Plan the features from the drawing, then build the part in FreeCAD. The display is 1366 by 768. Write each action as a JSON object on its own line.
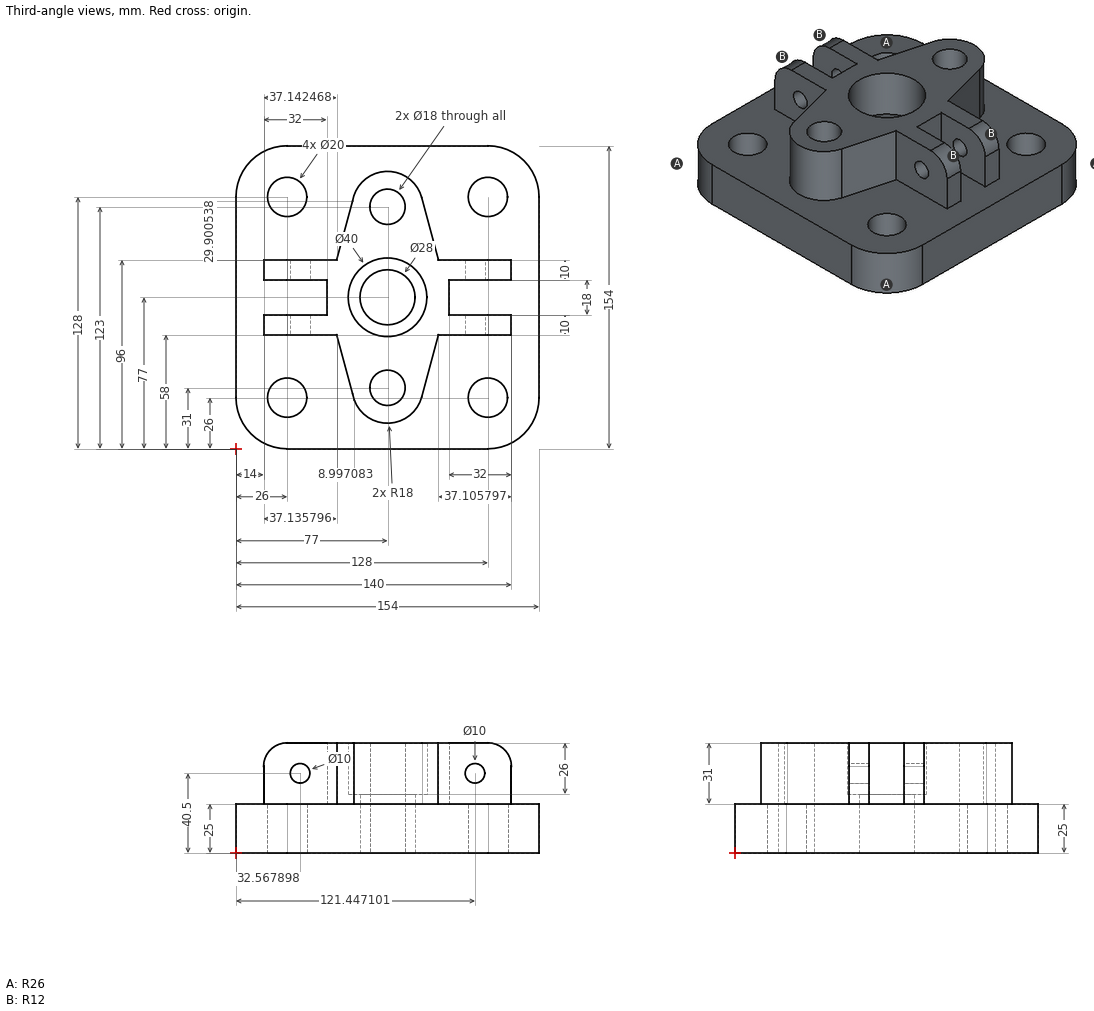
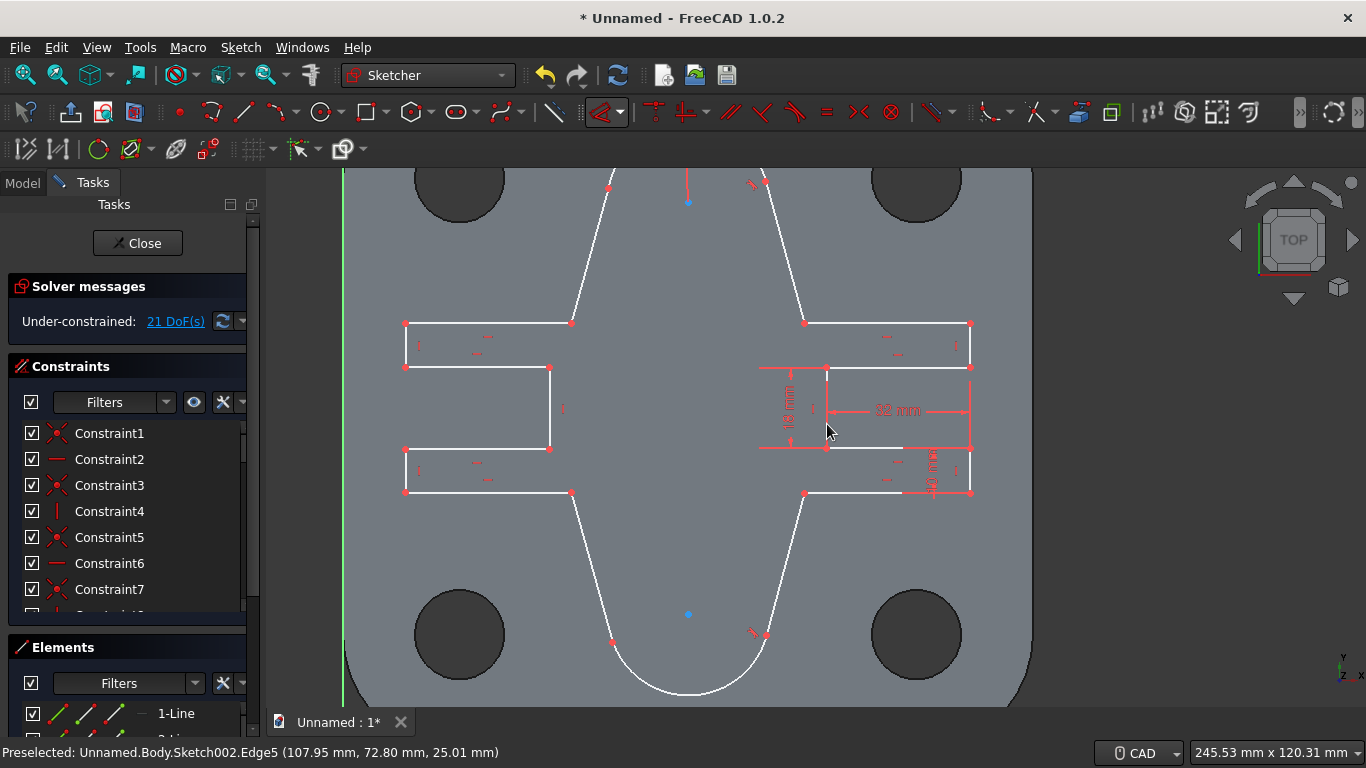
{"action": "left_click", "coordinate": [870, 368]}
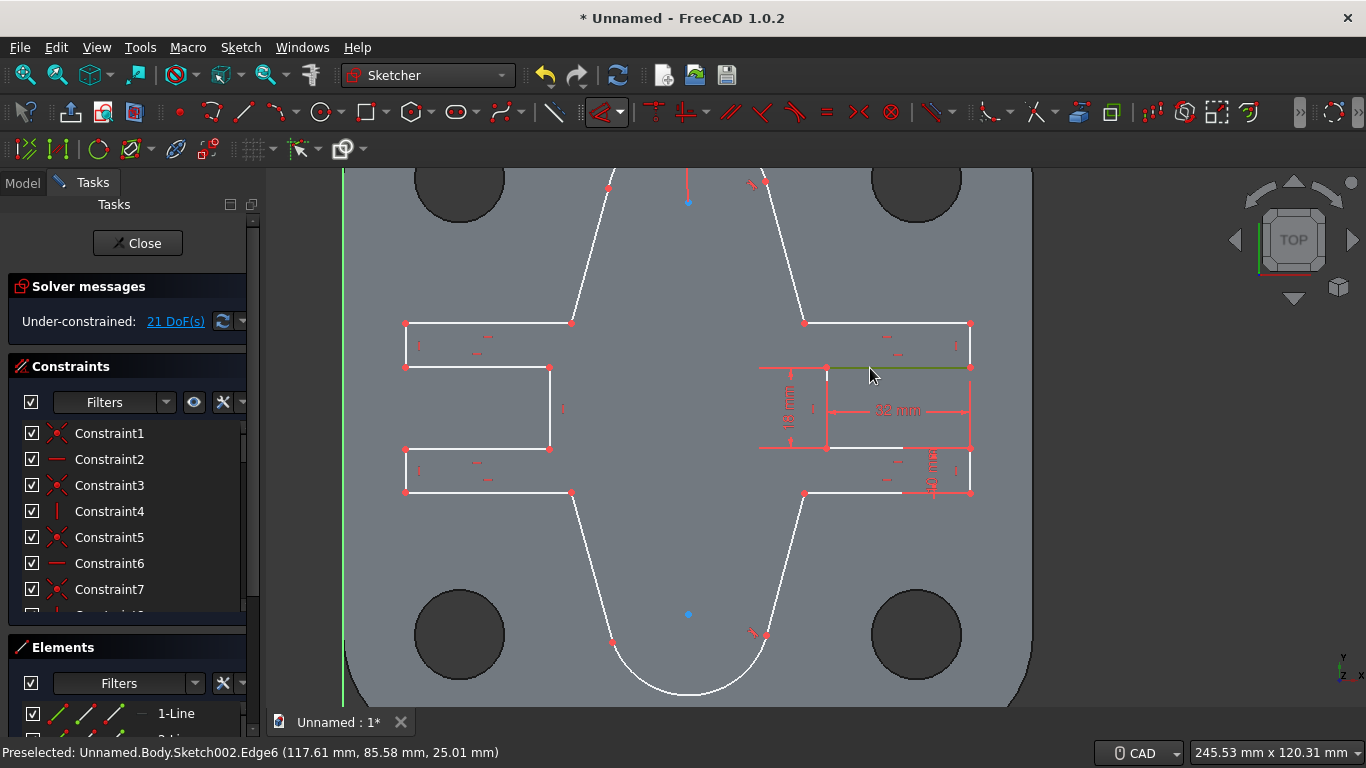
{"action": "key", "text": "l"}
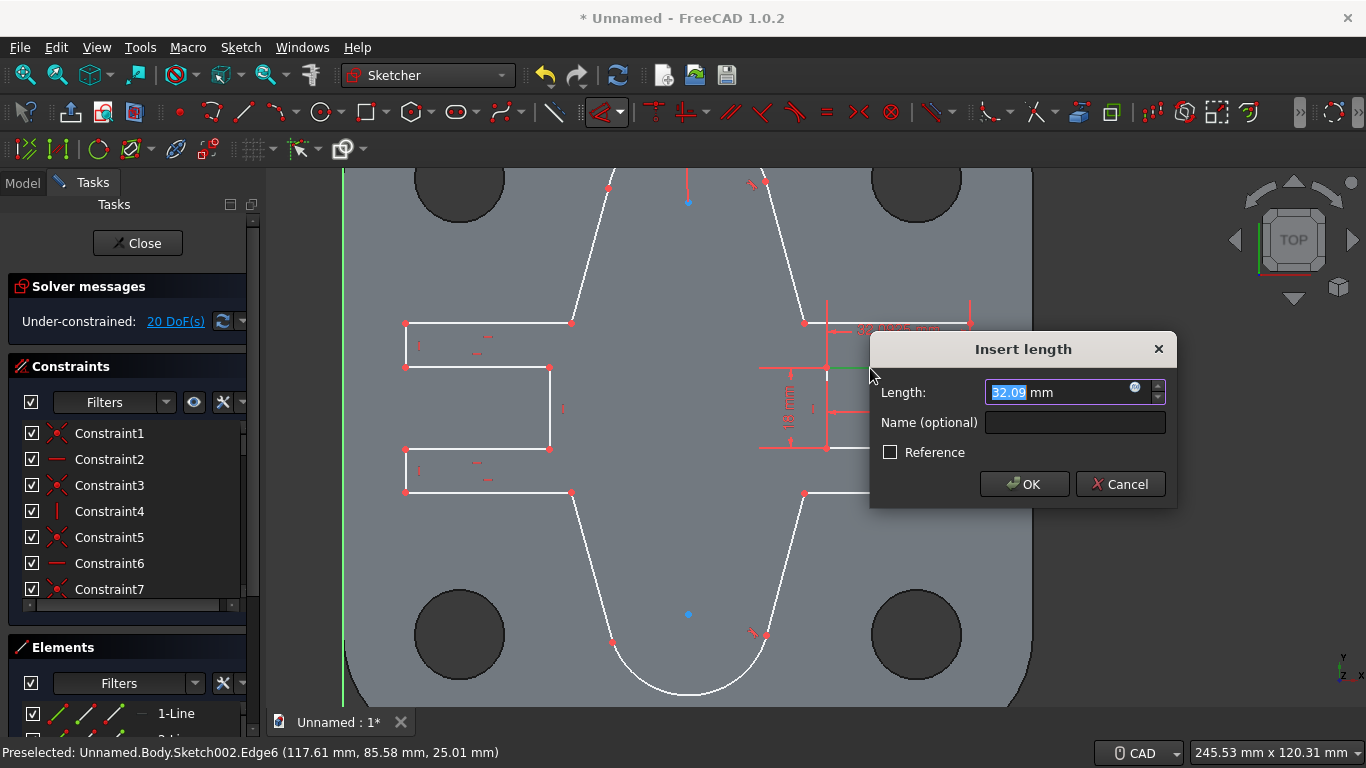
{"action": "type", "text": "32"}
{"action": "key", "text": "Return"}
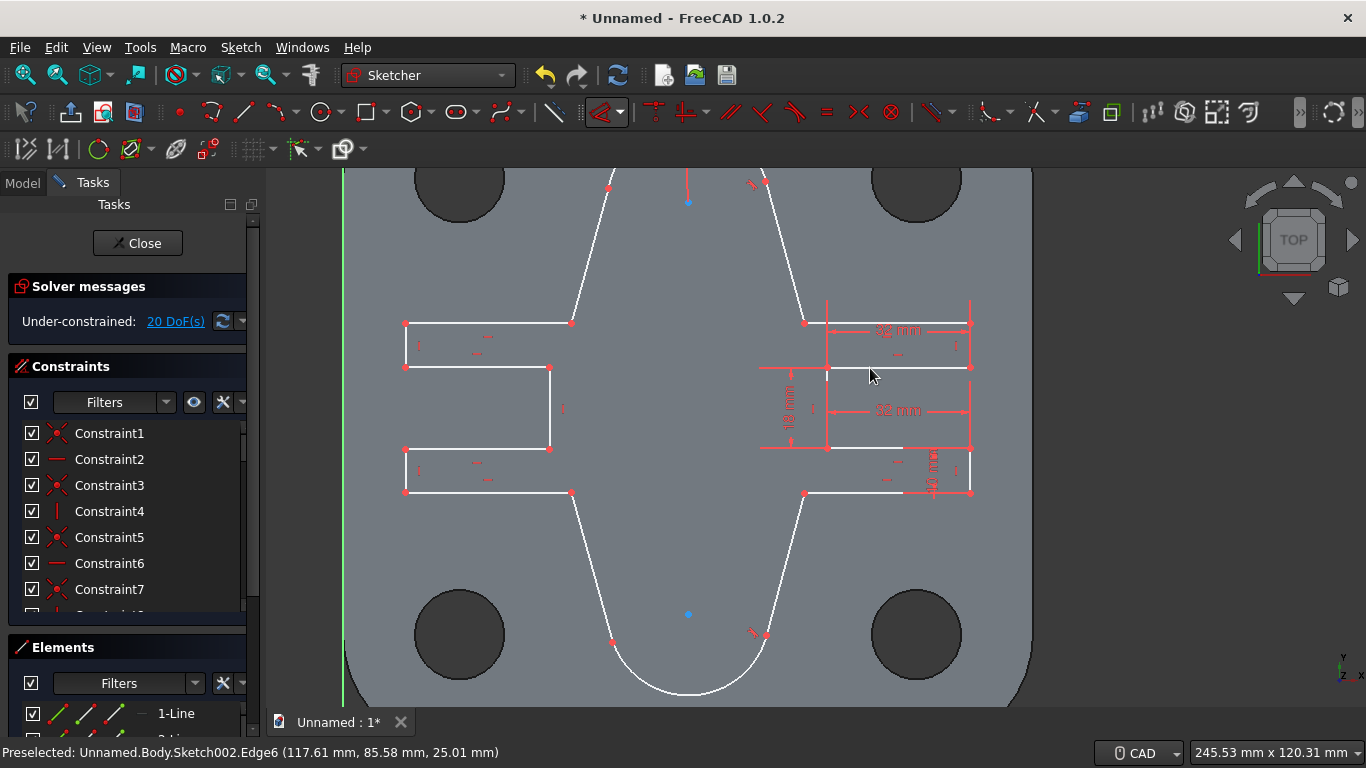
{"action": "left_click", "coordinate": [970, 354]}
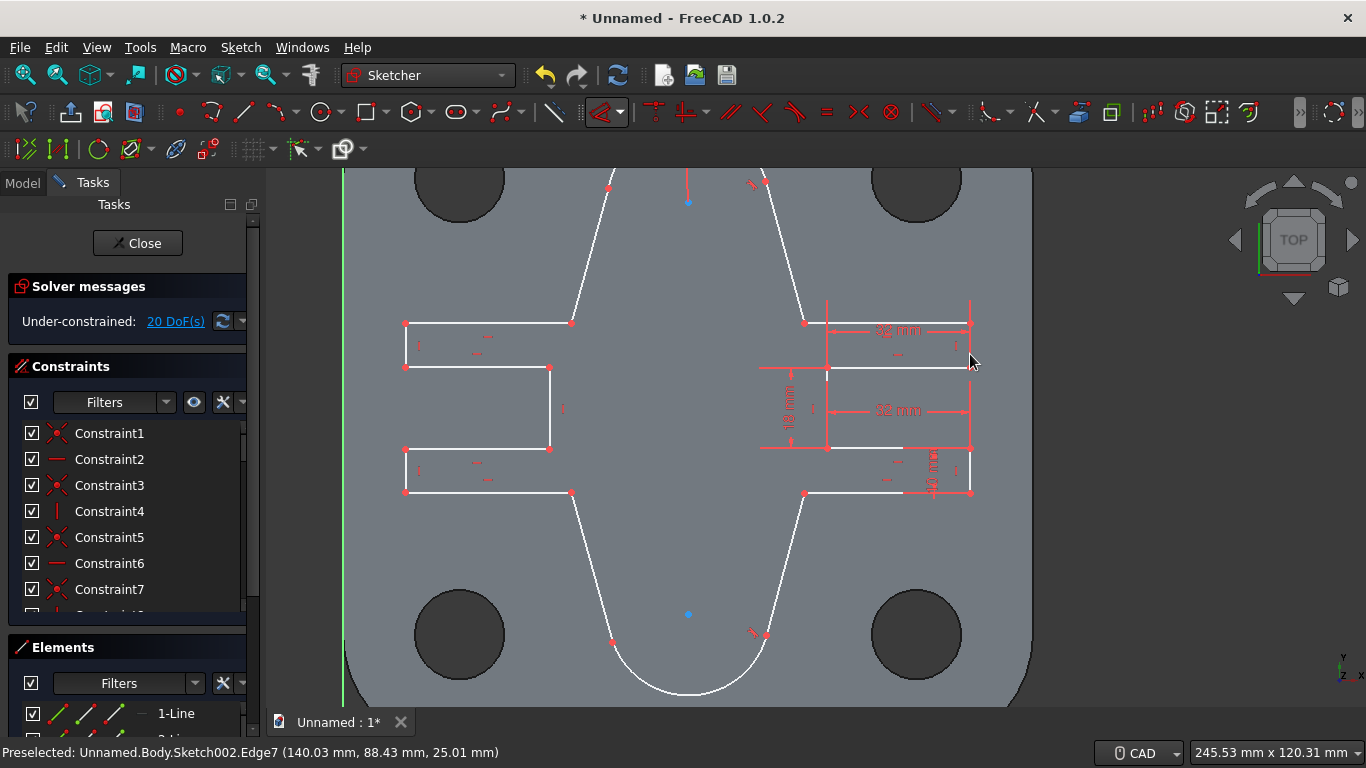
{"action": "key", "text": "i"}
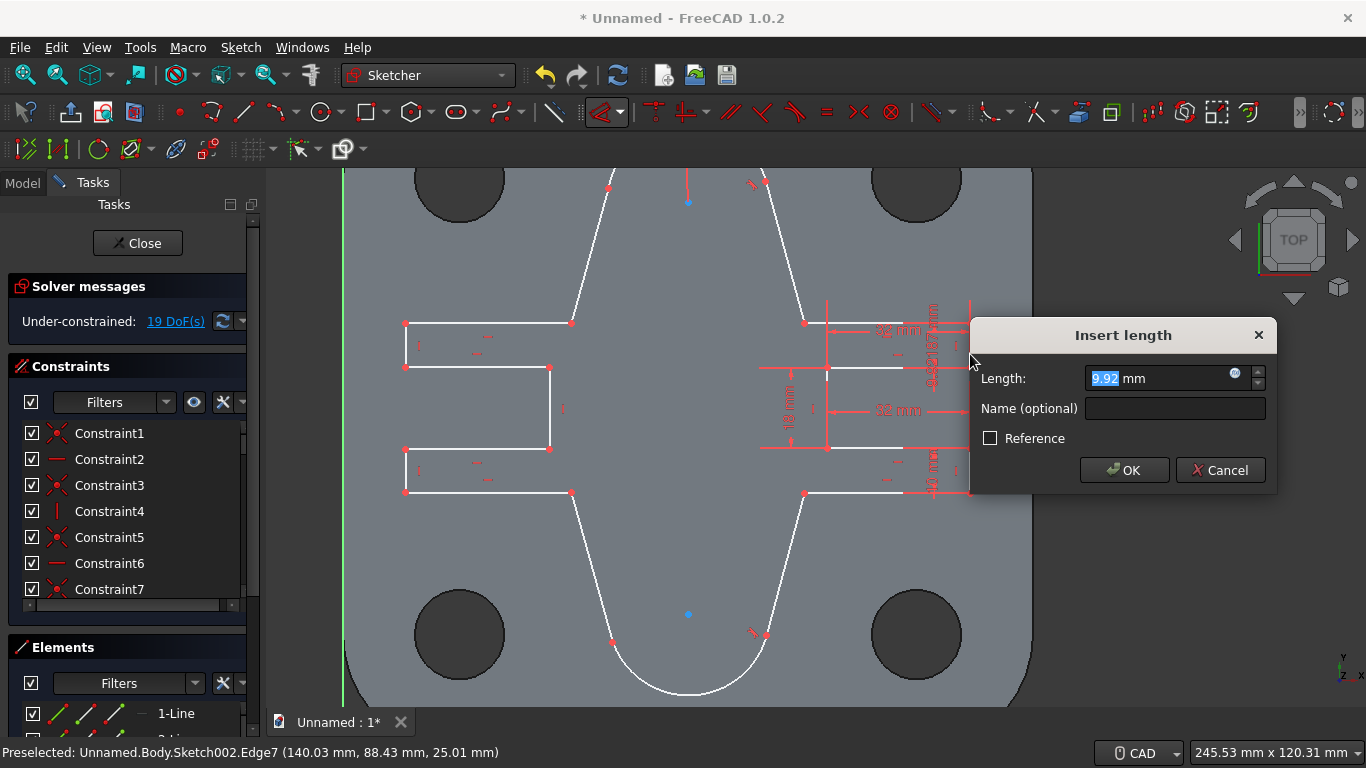
{"action": "type", "text": "10"}
{"action": "key", "text": "Return"}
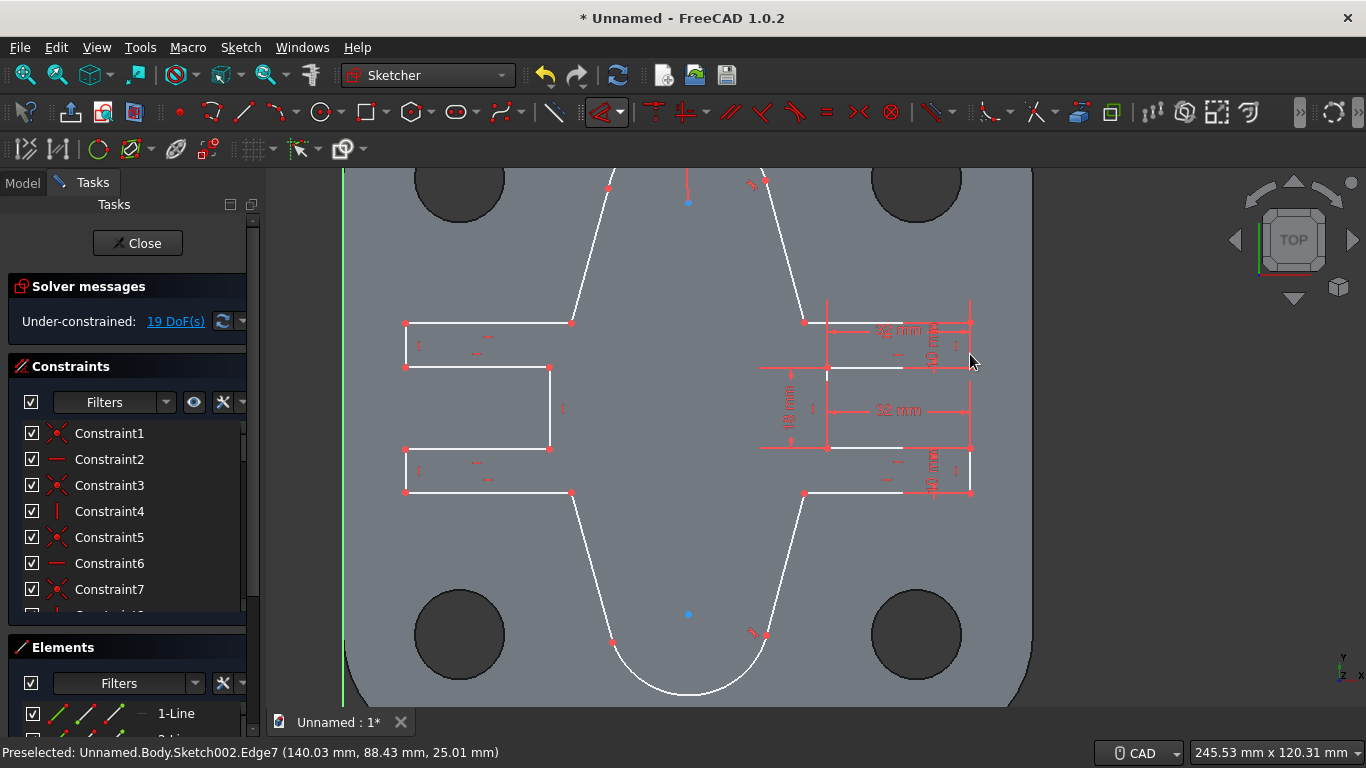
{"action": "left_click", "coordinate": [406, 336]}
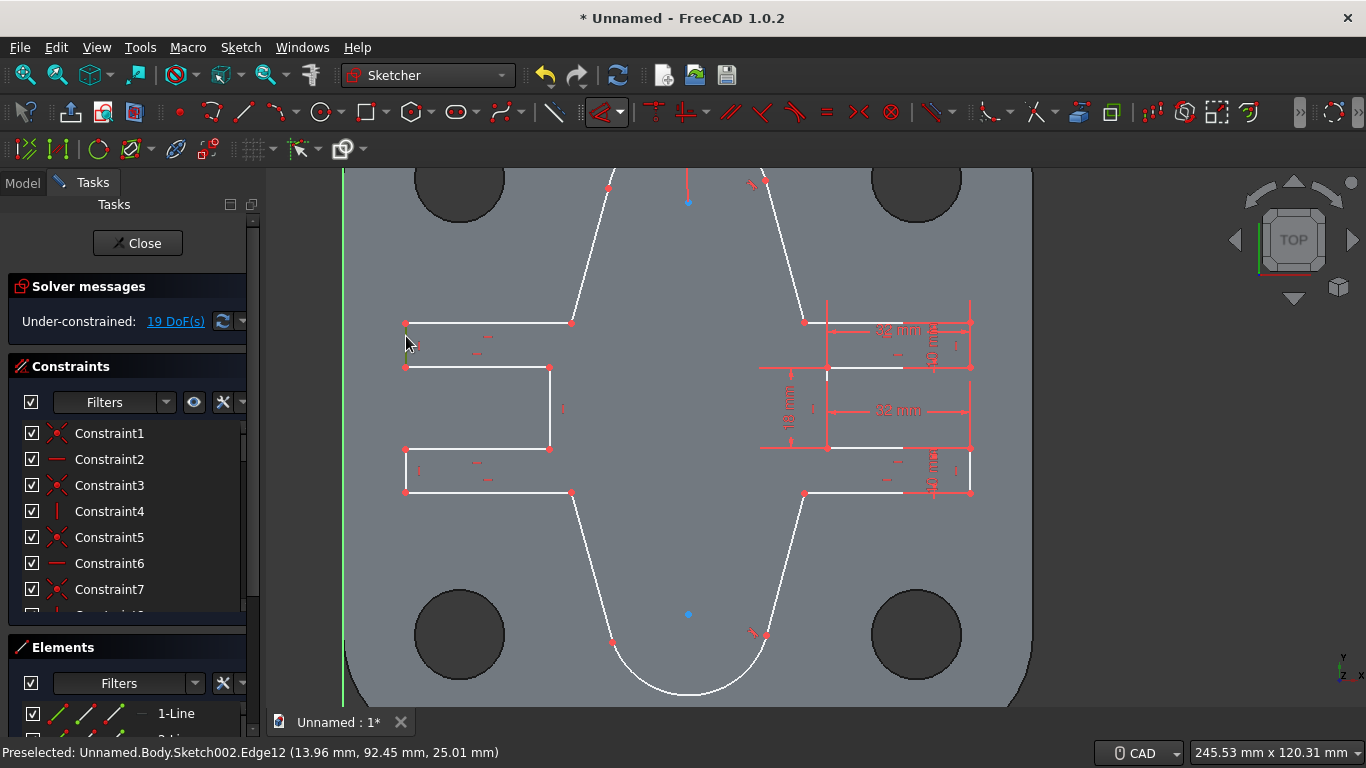
{"action": "left_click", "coordinate": [622, 112]}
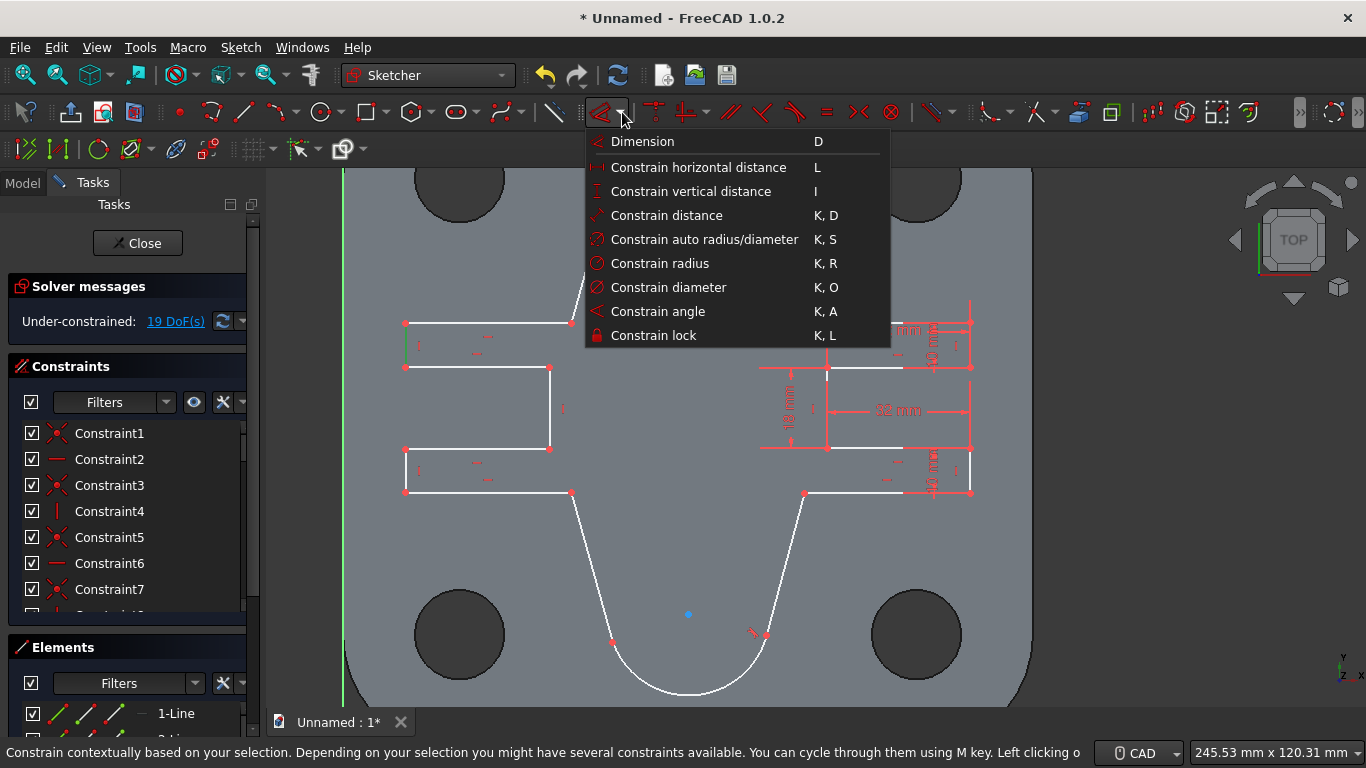
{"action": "left_click", "coordinate": [738, 191]}